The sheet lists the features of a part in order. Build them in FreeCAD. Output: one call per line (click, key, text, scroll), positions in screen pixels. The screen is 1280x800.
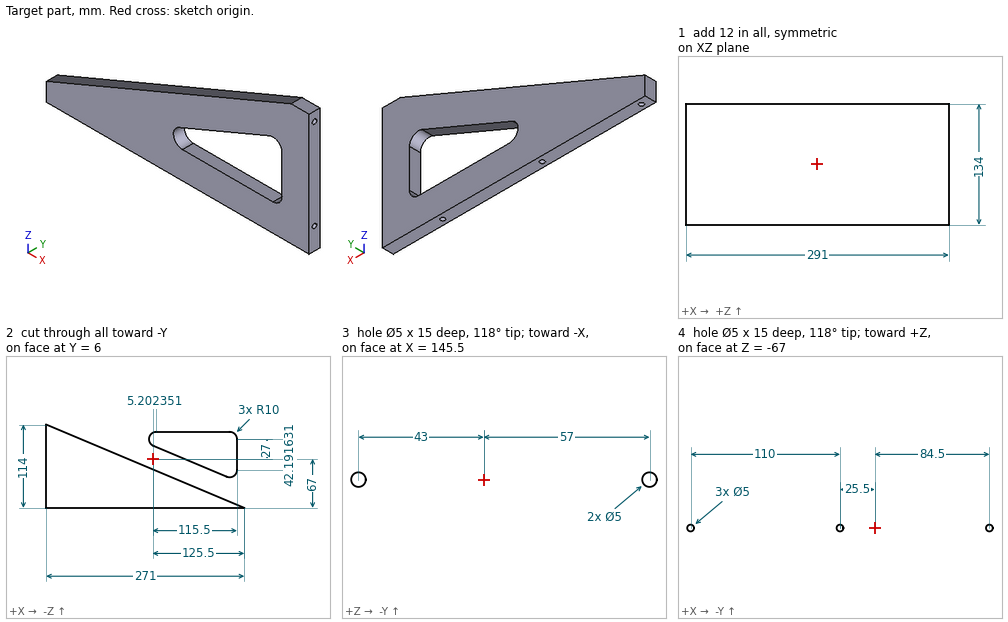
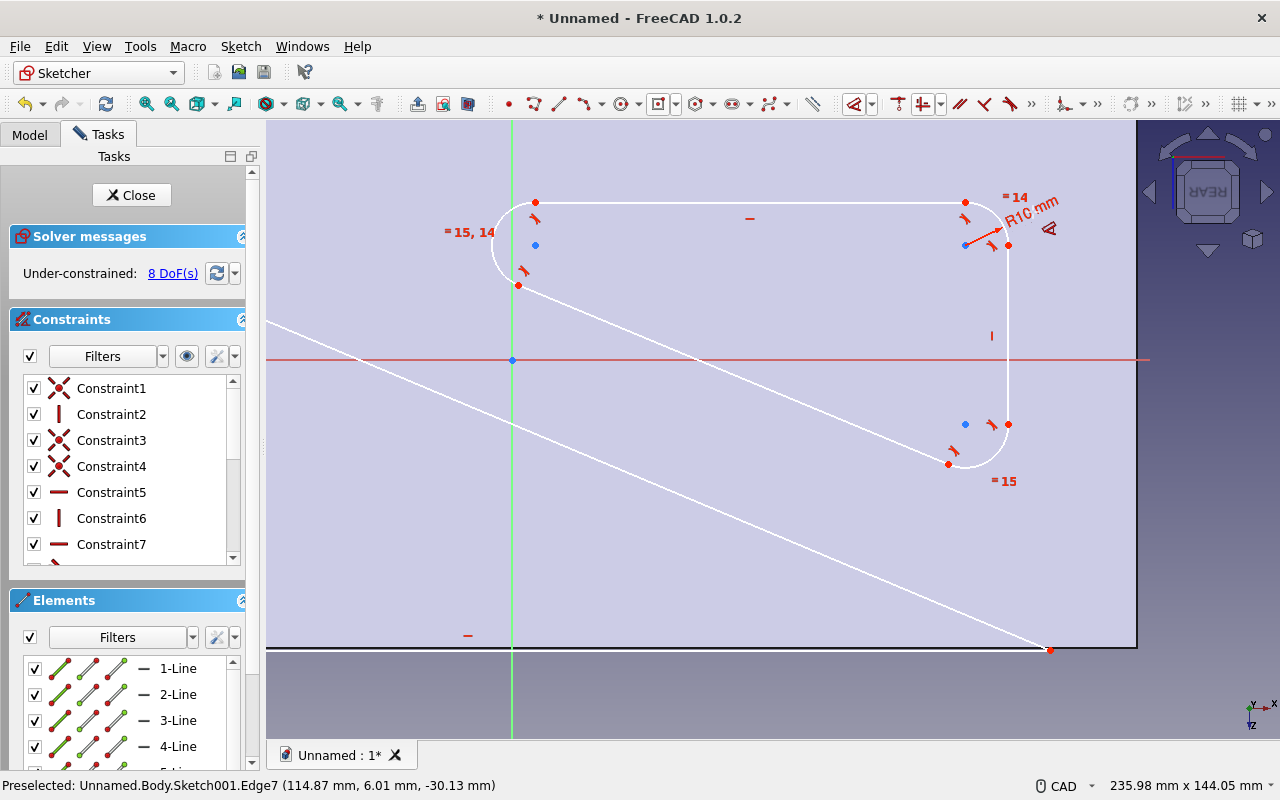
scroll(991, 461, down, 3)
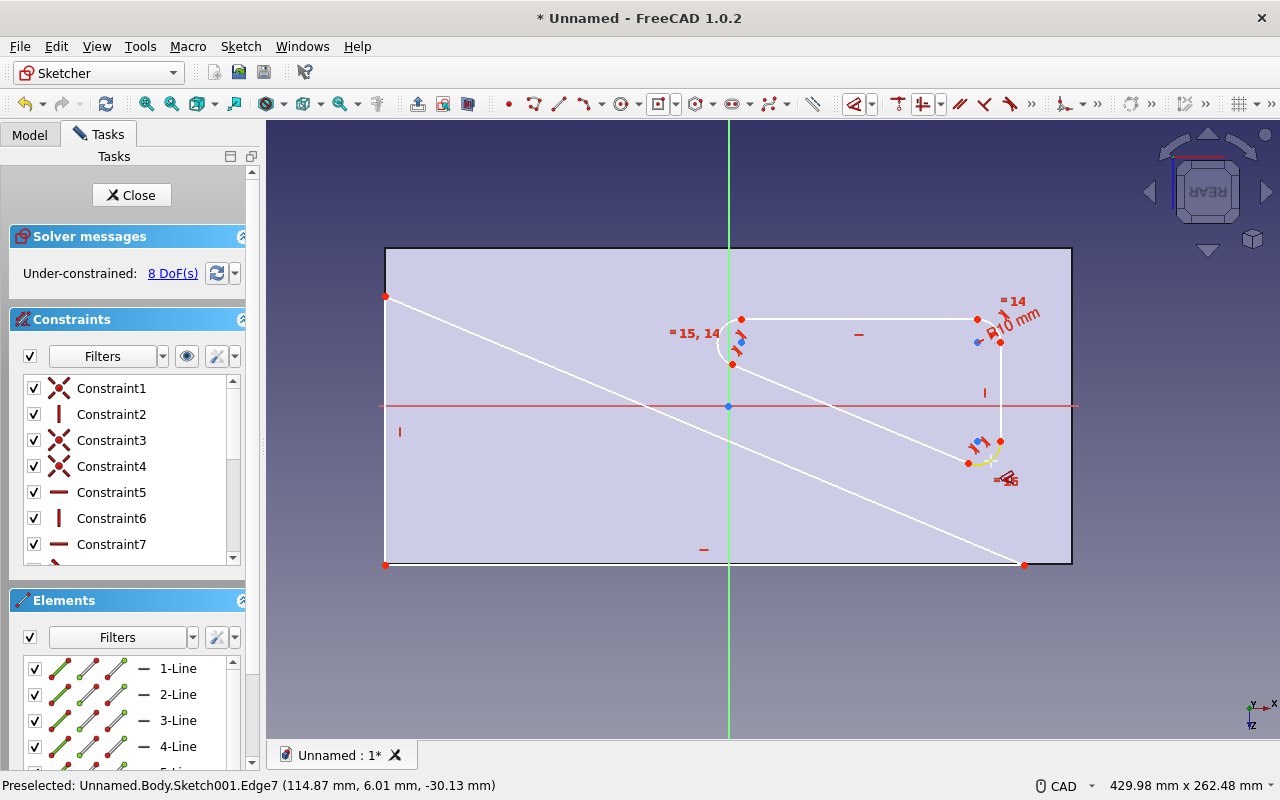
click(385, 377)
click(351, 431)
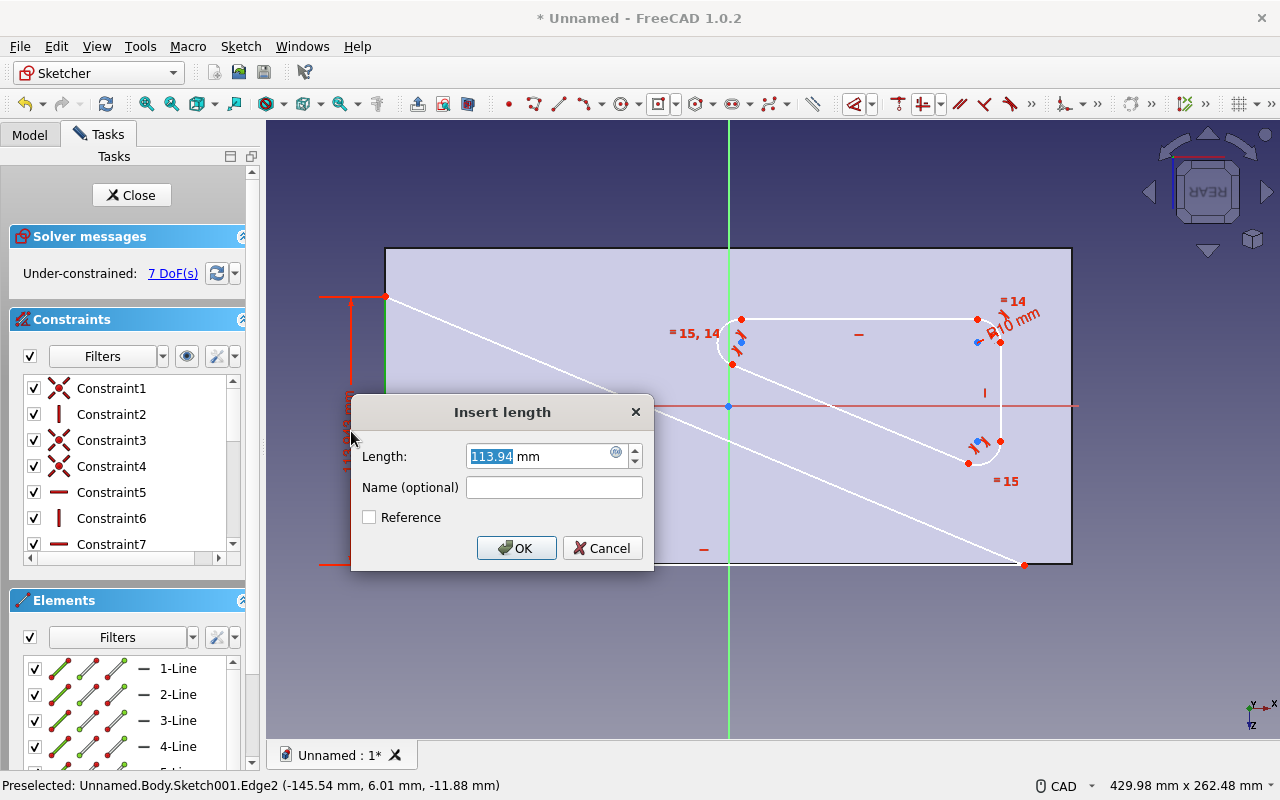
text(114)
key(Return)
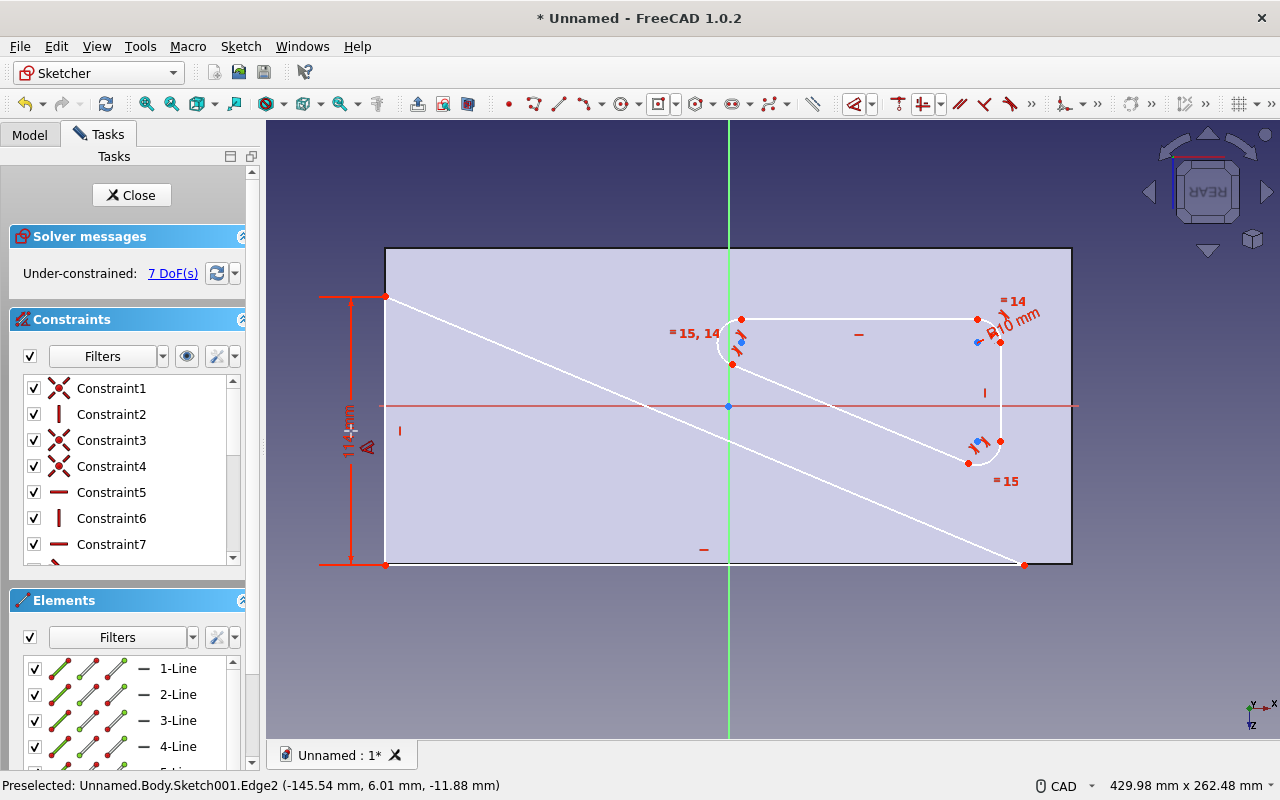
click(577, 565)
click(705, 599)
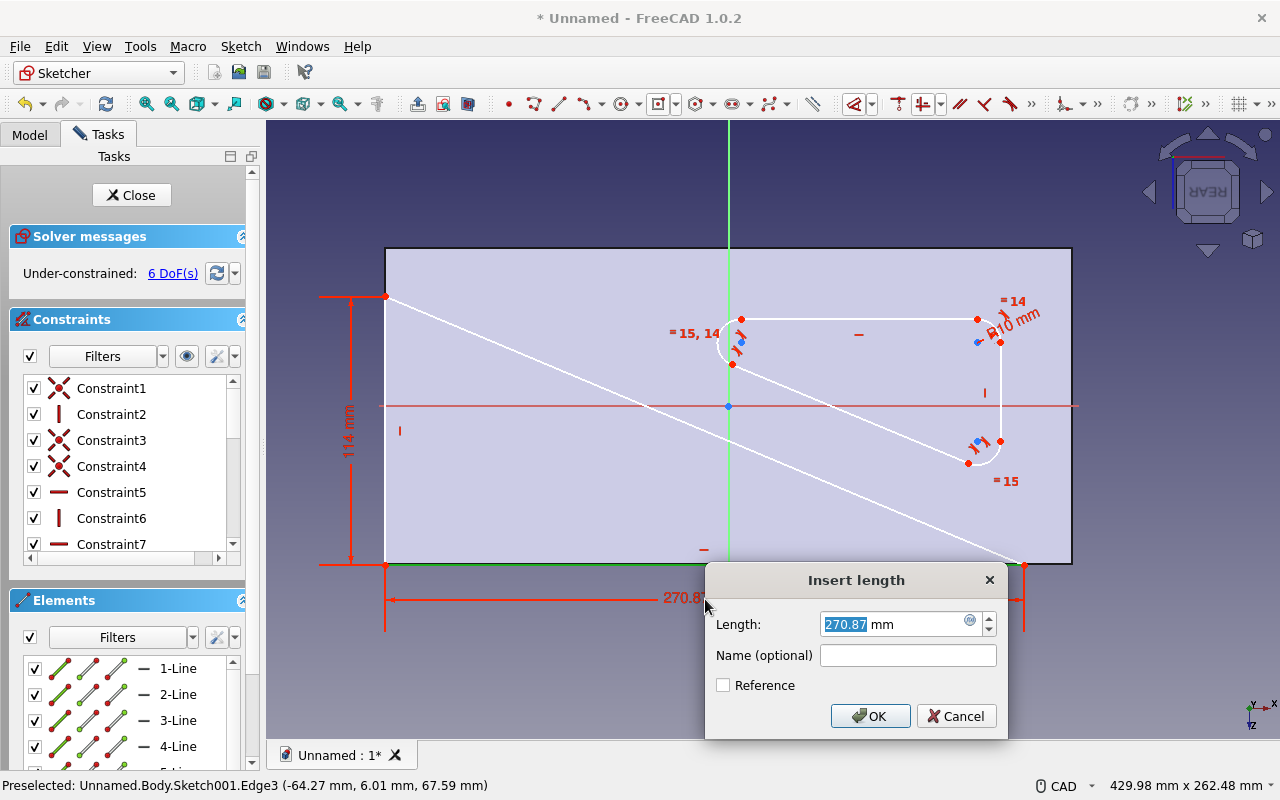
text(271)
key(Return)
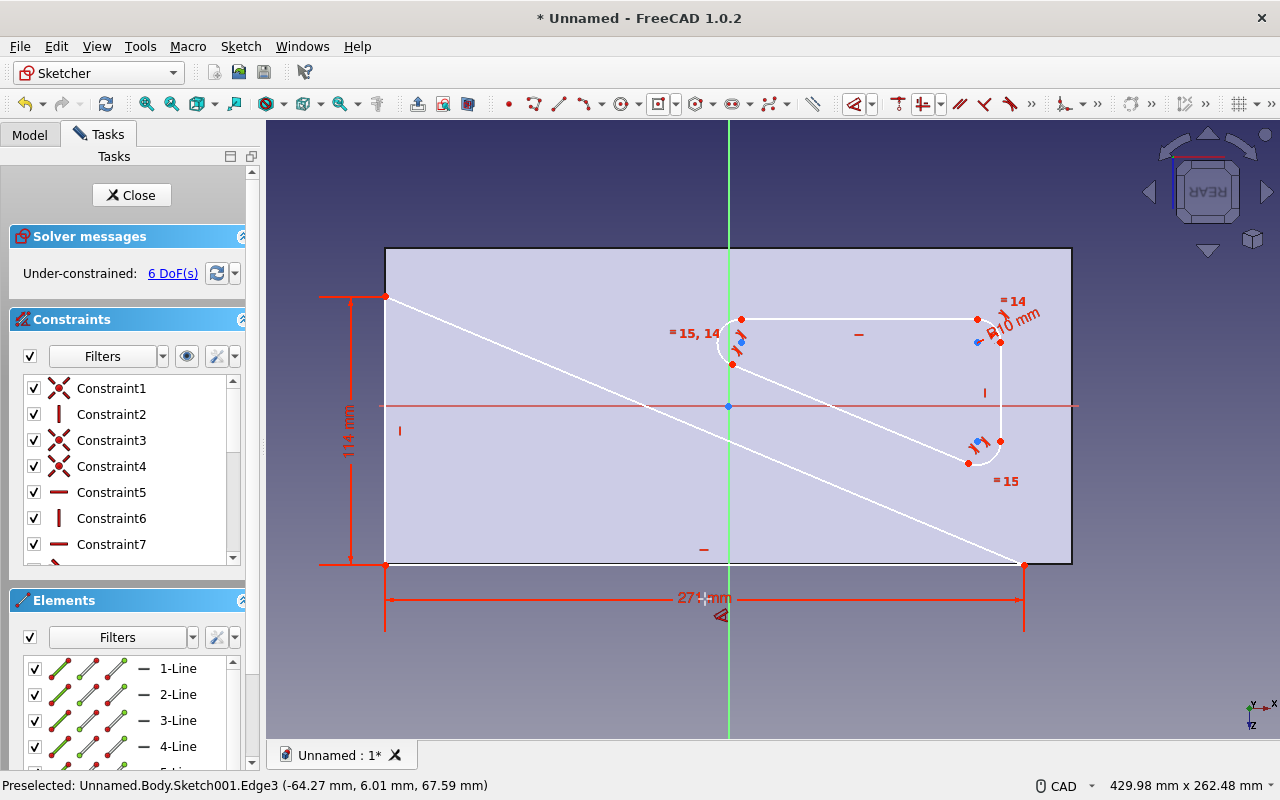
click(1024, 565)
click(1058, 486)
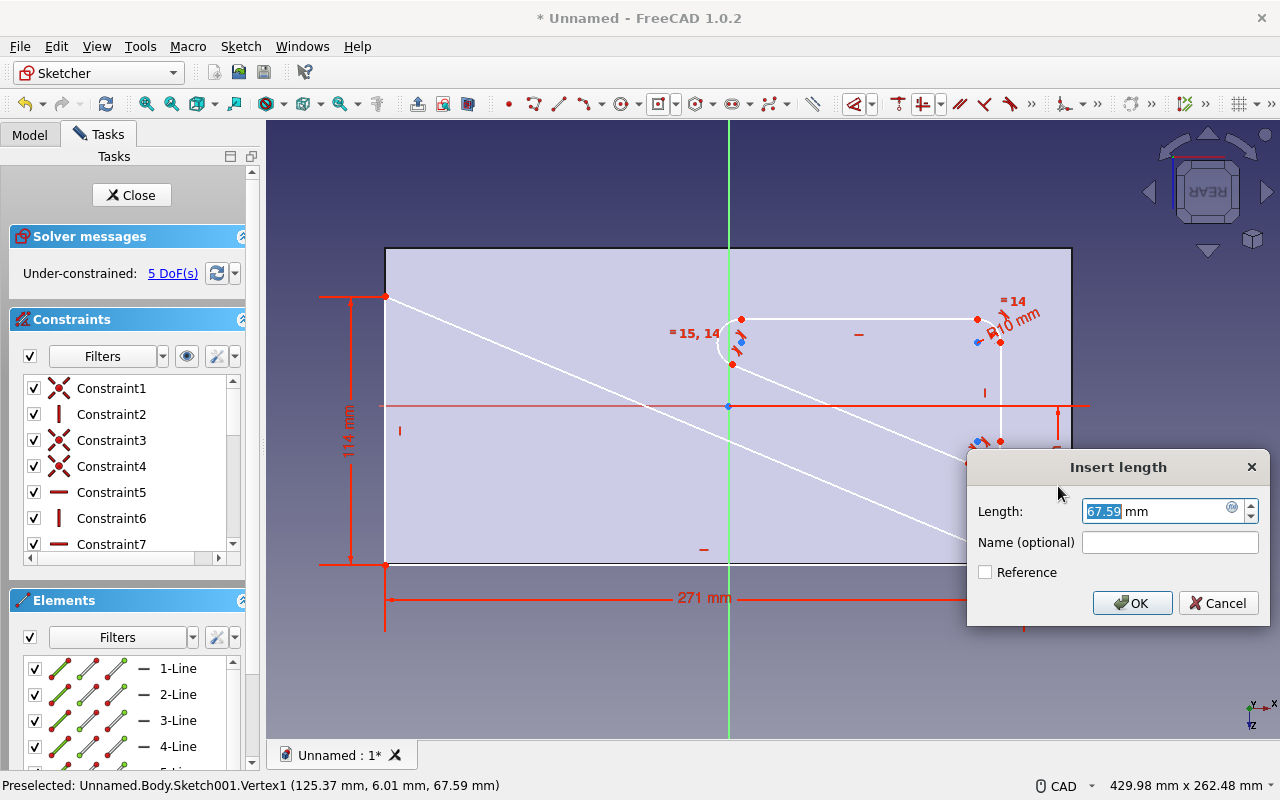
text(67)
key(Return)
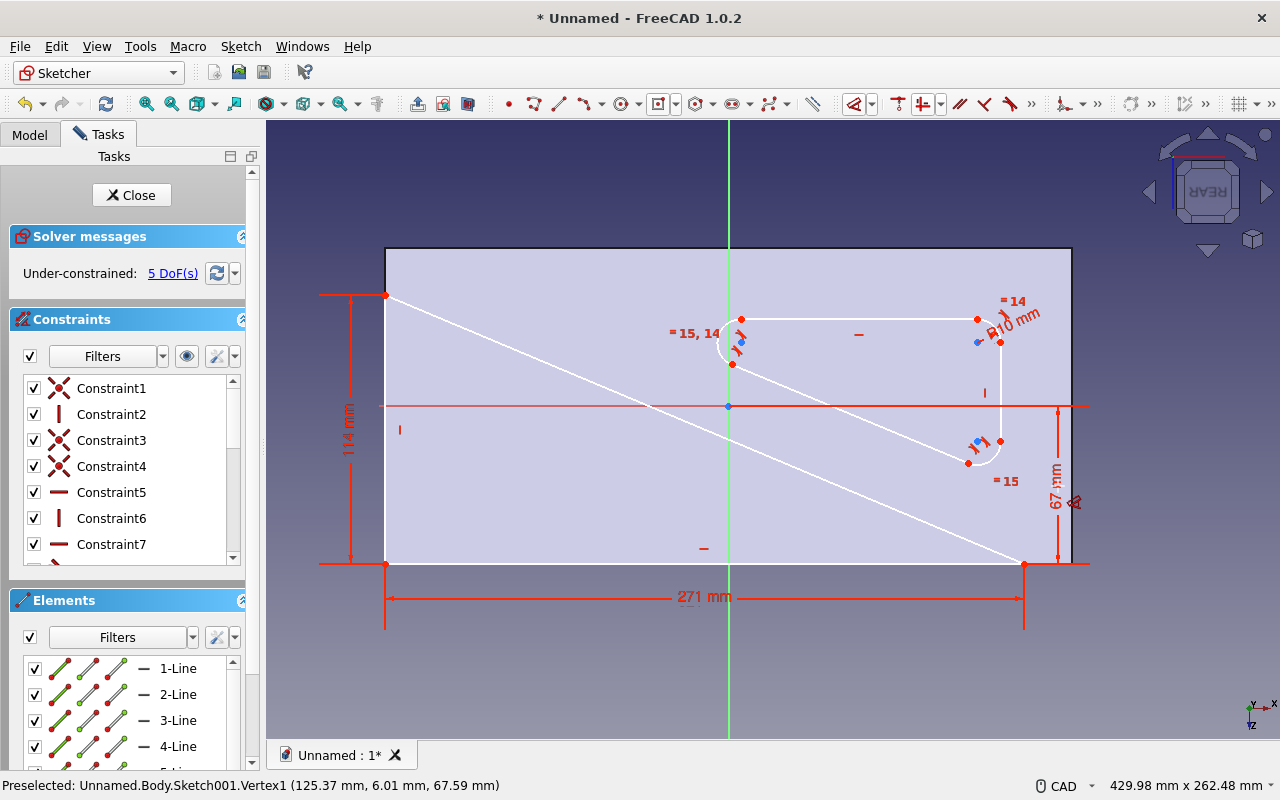
click(1001, 343)
click(1035, 374)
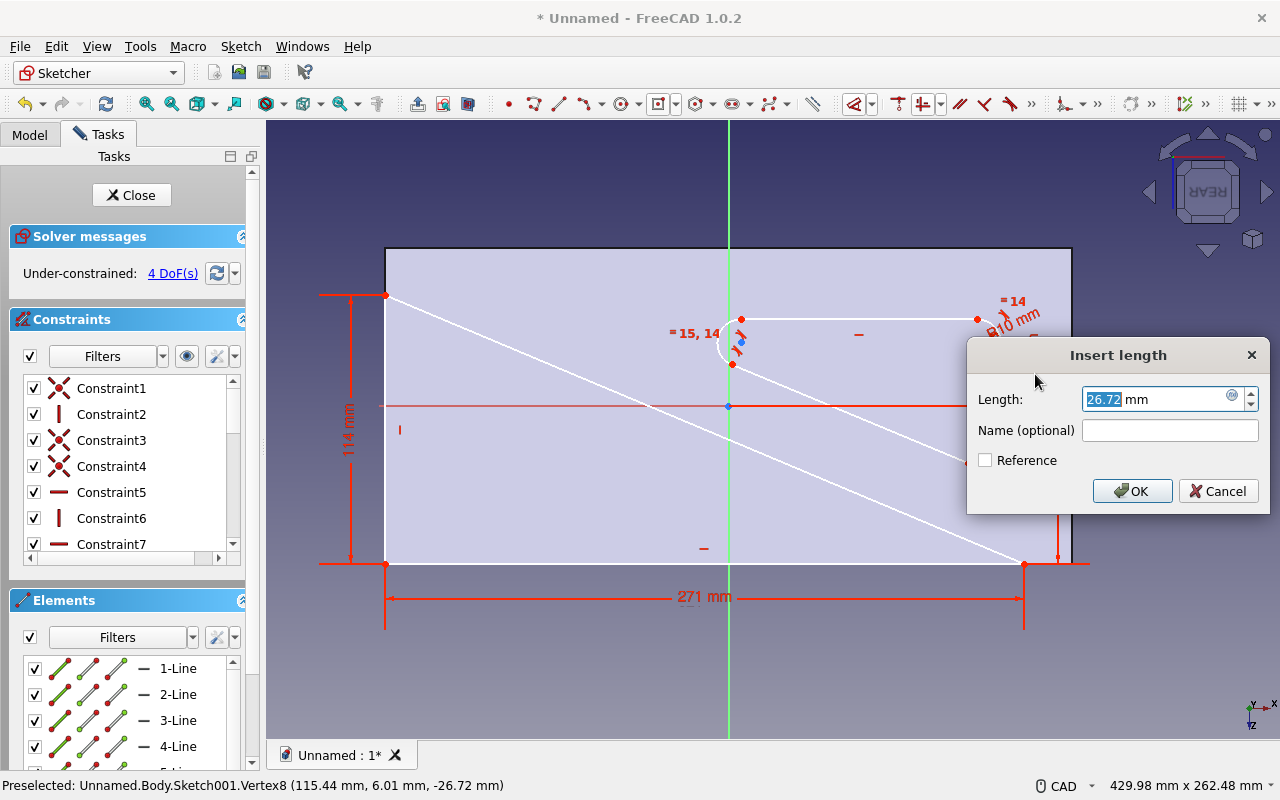
text(27)
key(Return)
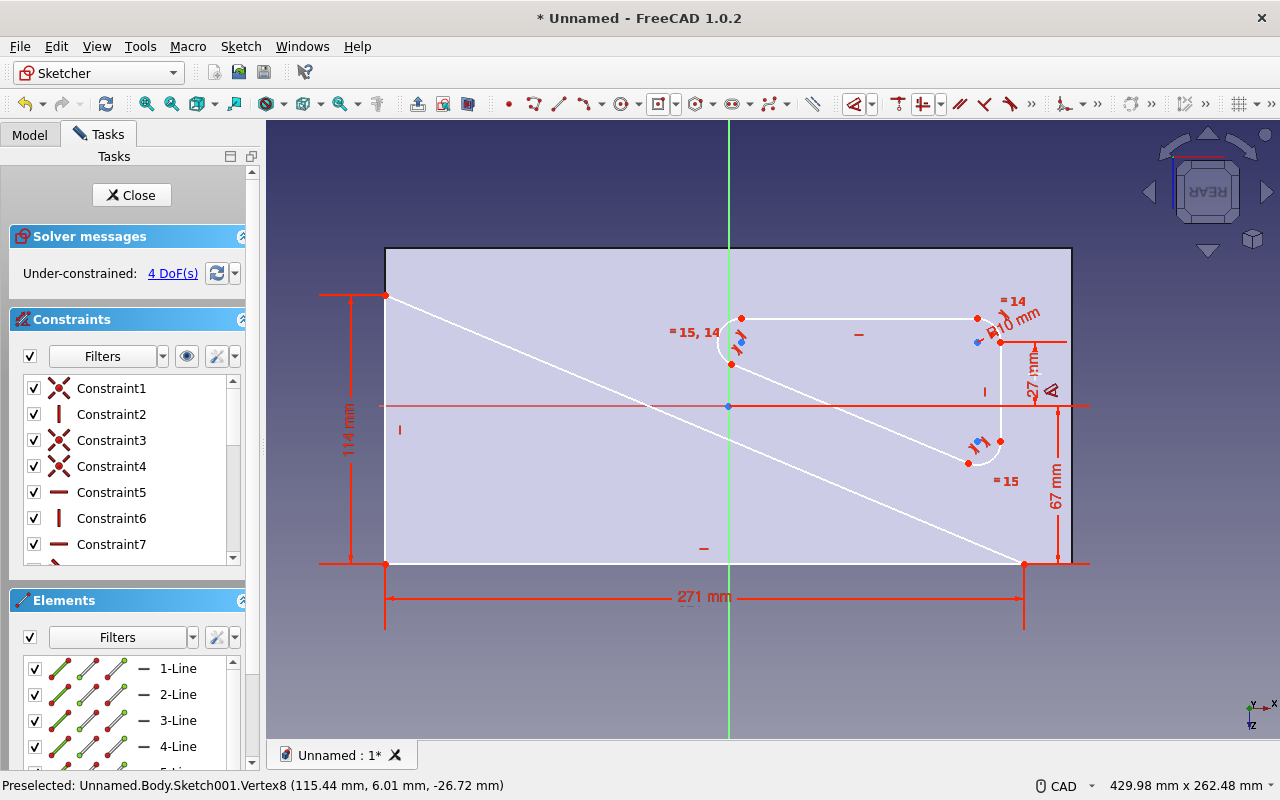
click(1024, 564)
click(876, 598)